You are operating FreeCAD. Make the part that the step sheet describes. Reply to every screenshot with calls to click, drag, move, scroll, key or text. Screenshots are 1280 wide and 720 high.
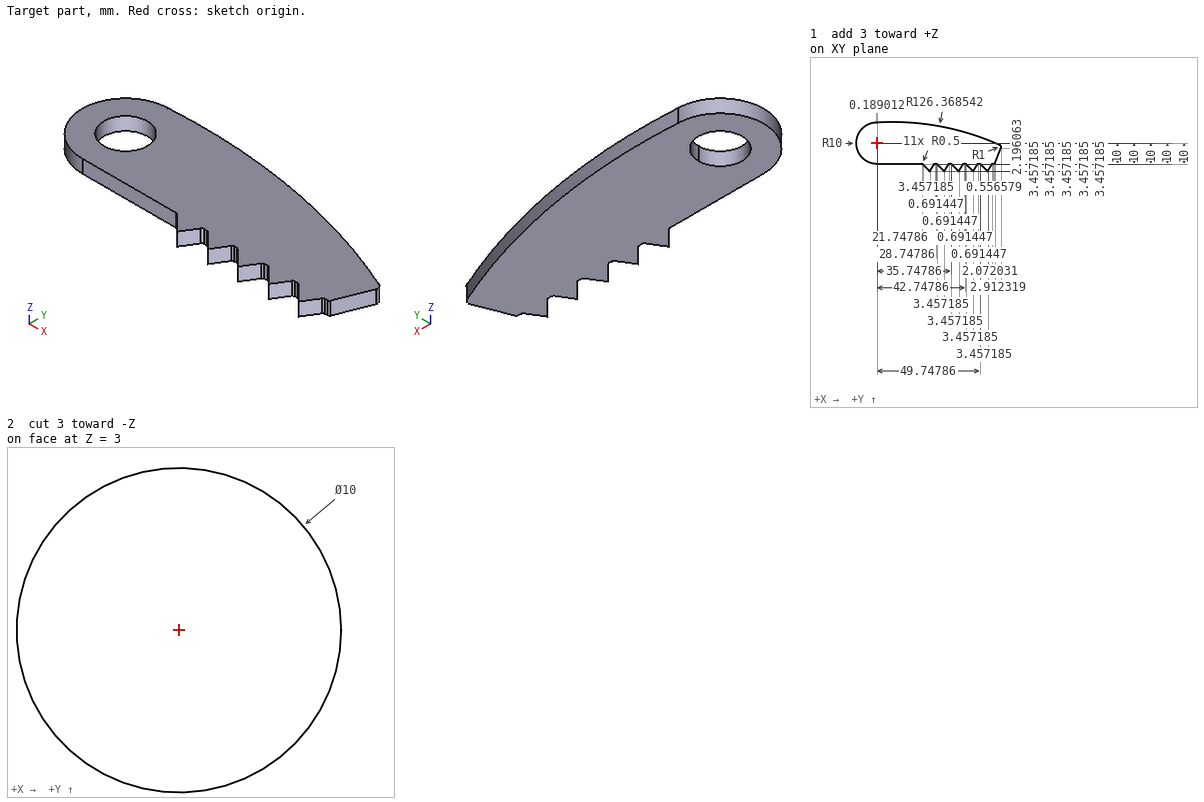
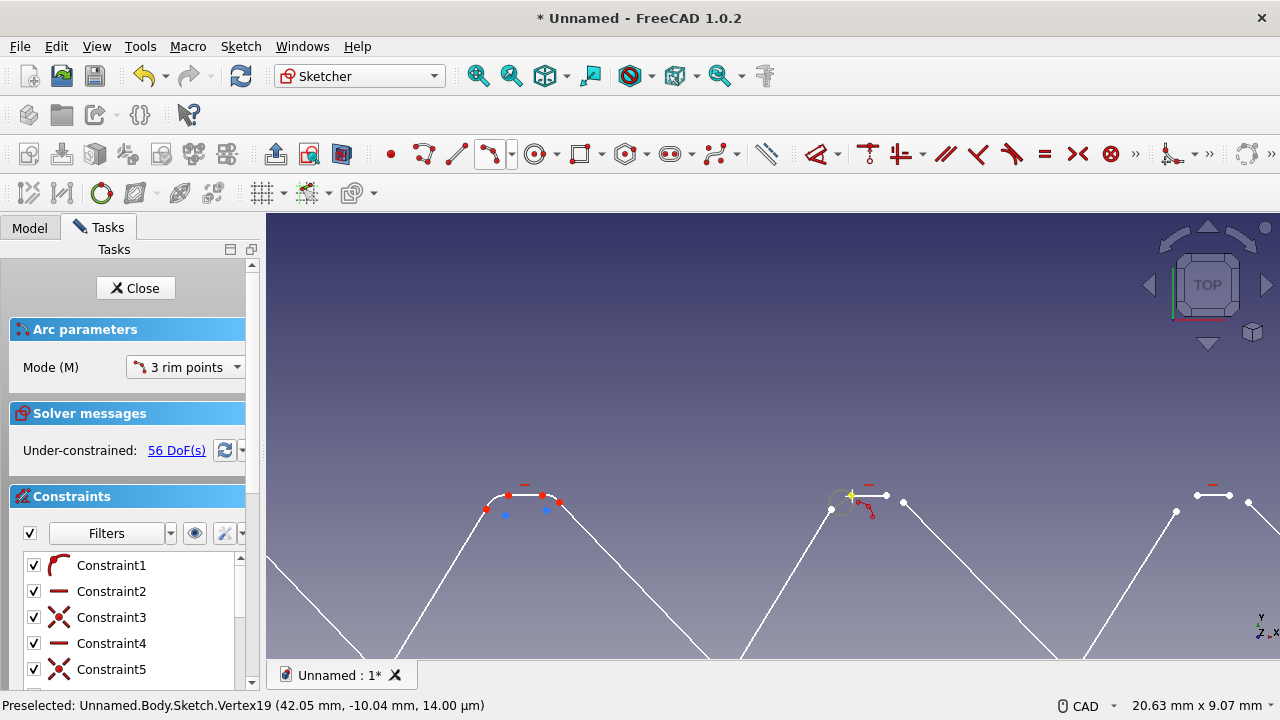
scroll(840, 497, up, 9)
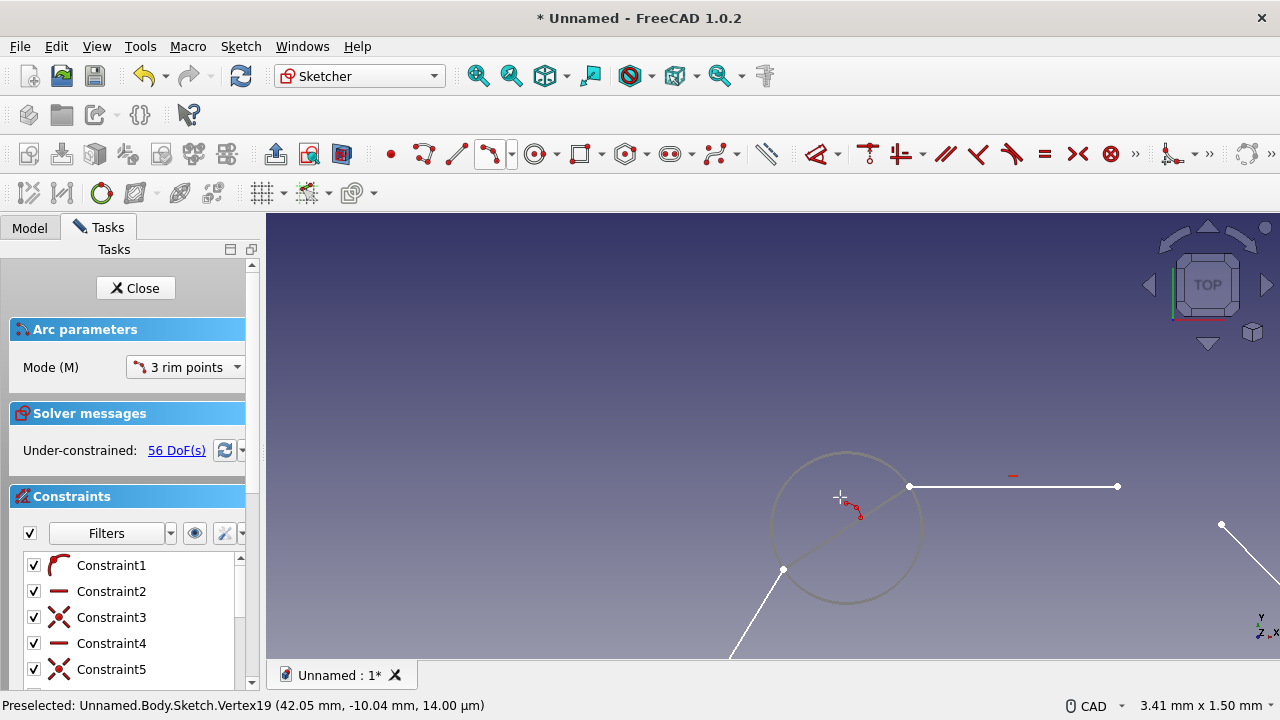
click(840, 495)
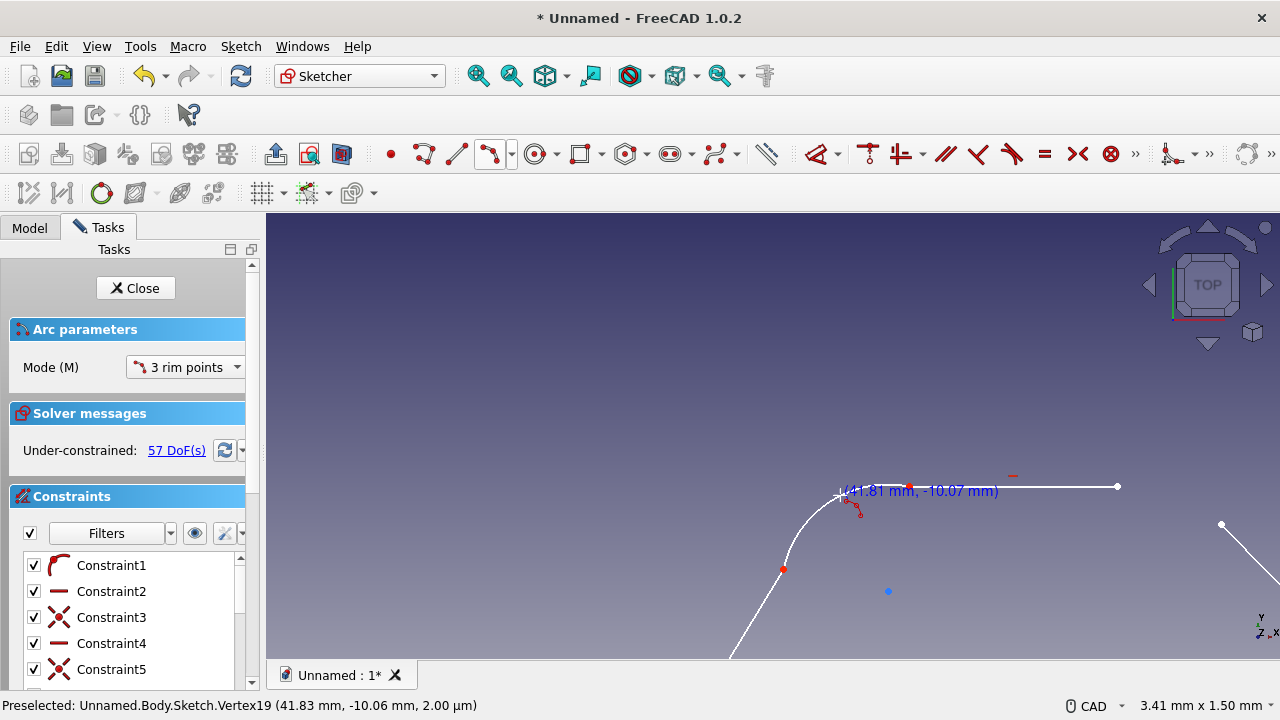
scroll(873, 519, down, 17)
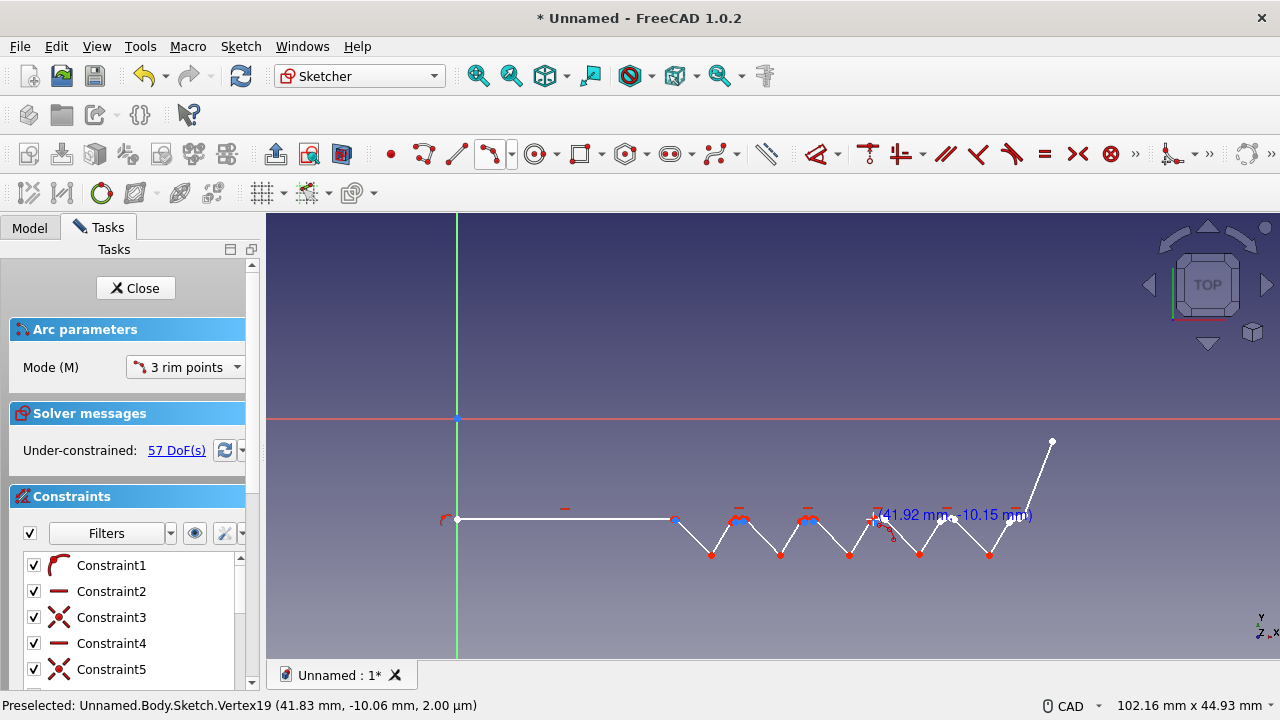
scroll(882, 518, up, 8)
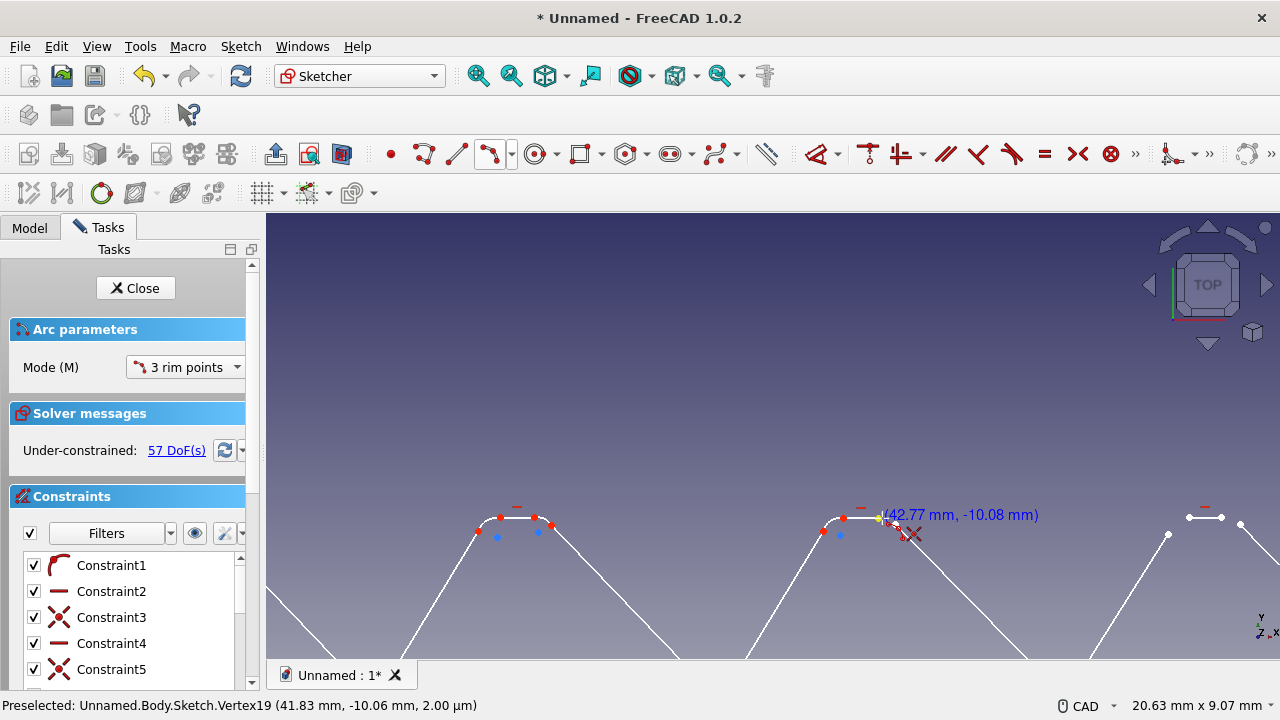
click(878, 518)
click(895, 524)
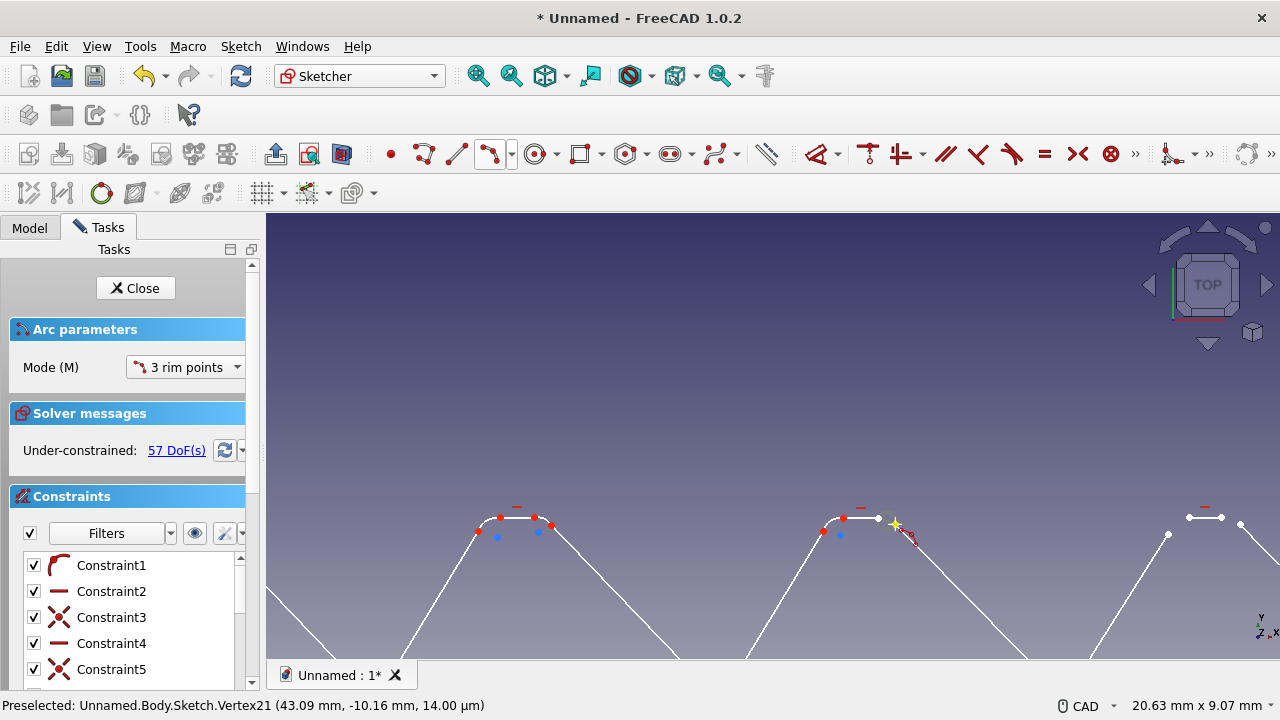
scroll(888, 518, up, 11)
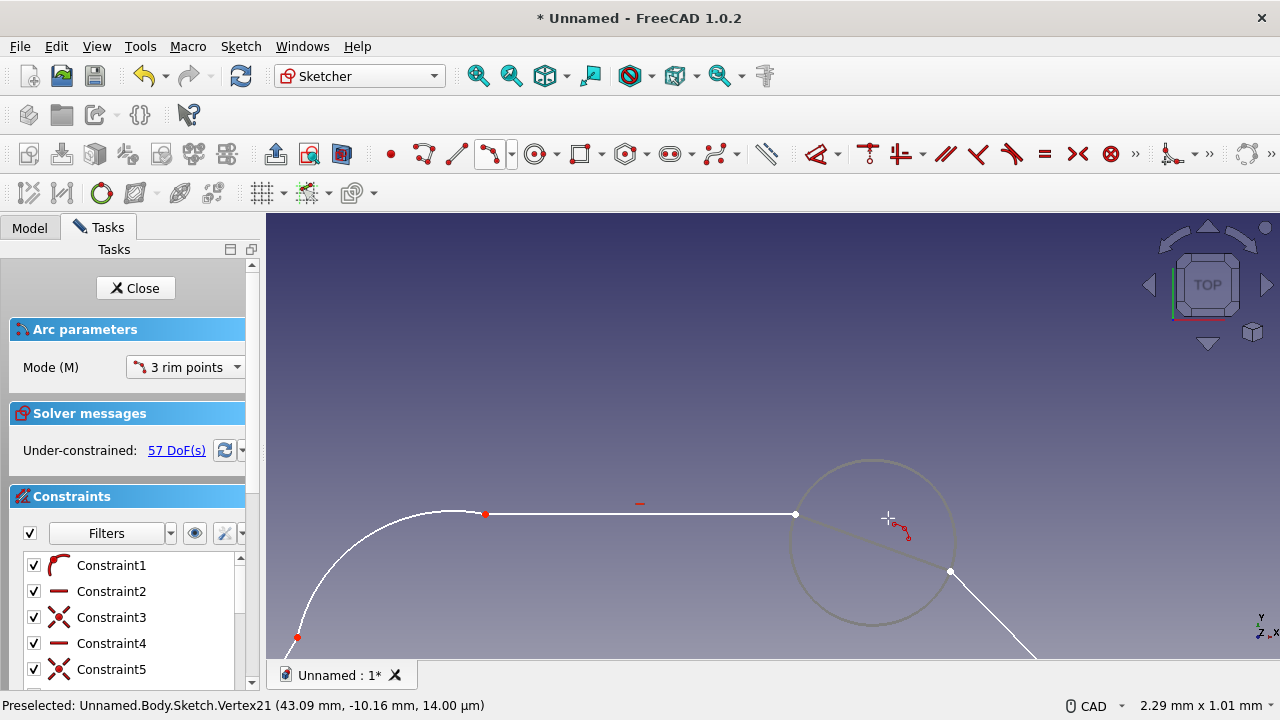
click(881, 516)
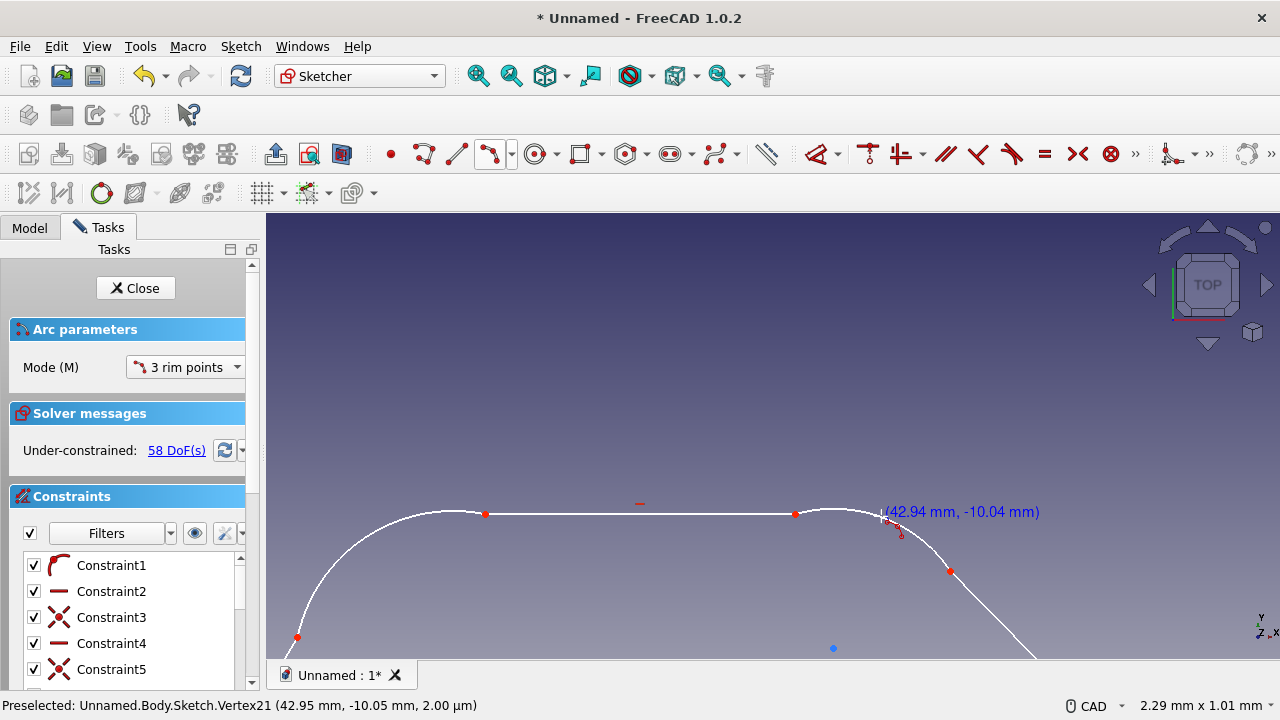
scroll(704, 436, down, 15)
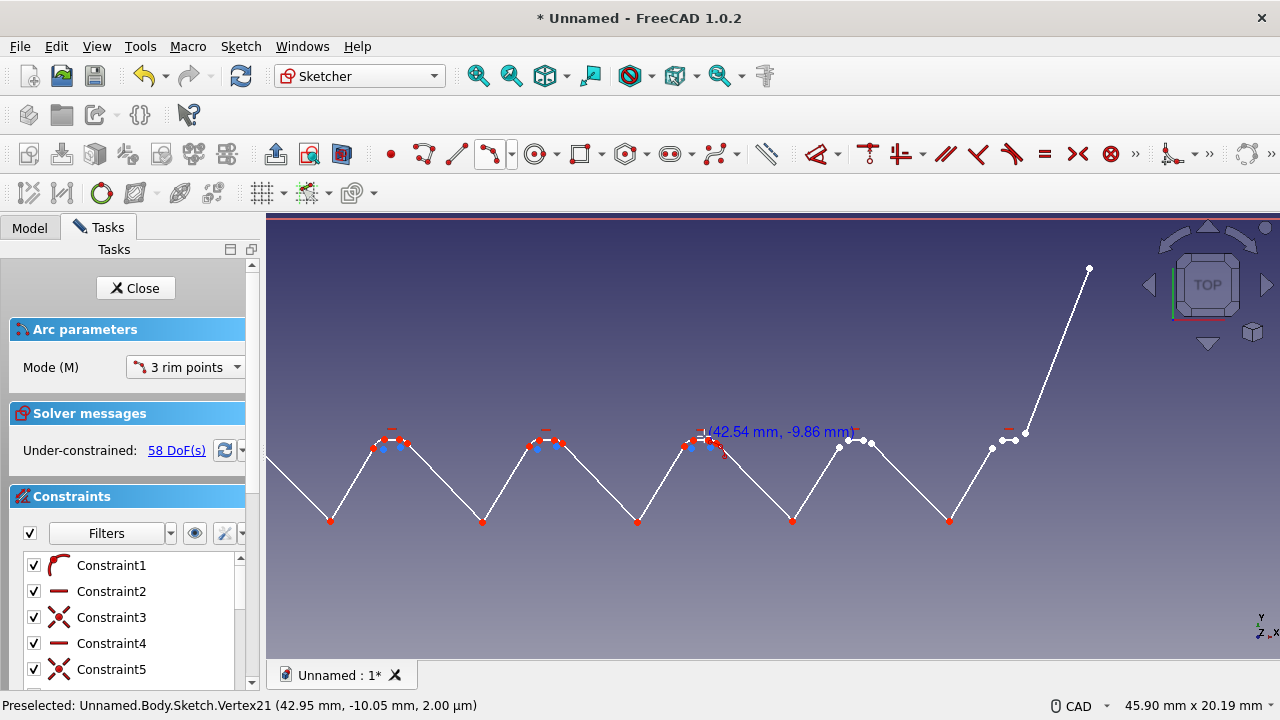
scroll(930, 539, down, 5)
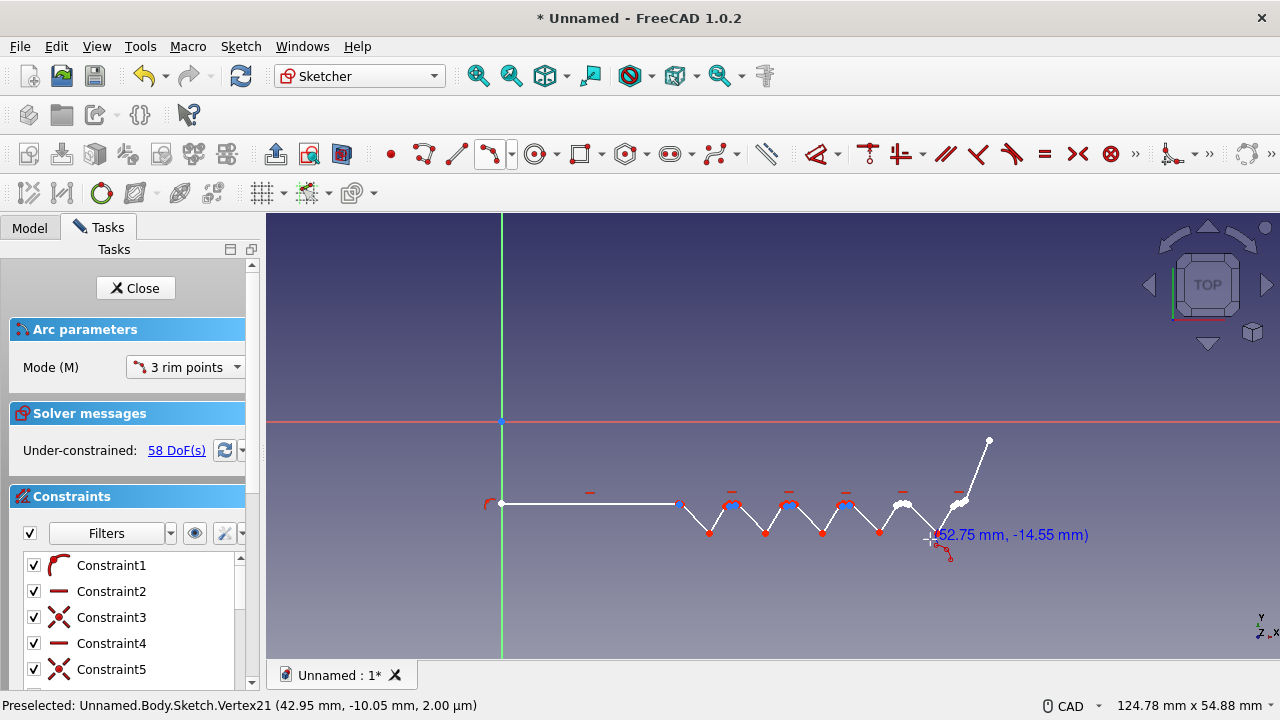
scroll(897, 505, up, 7)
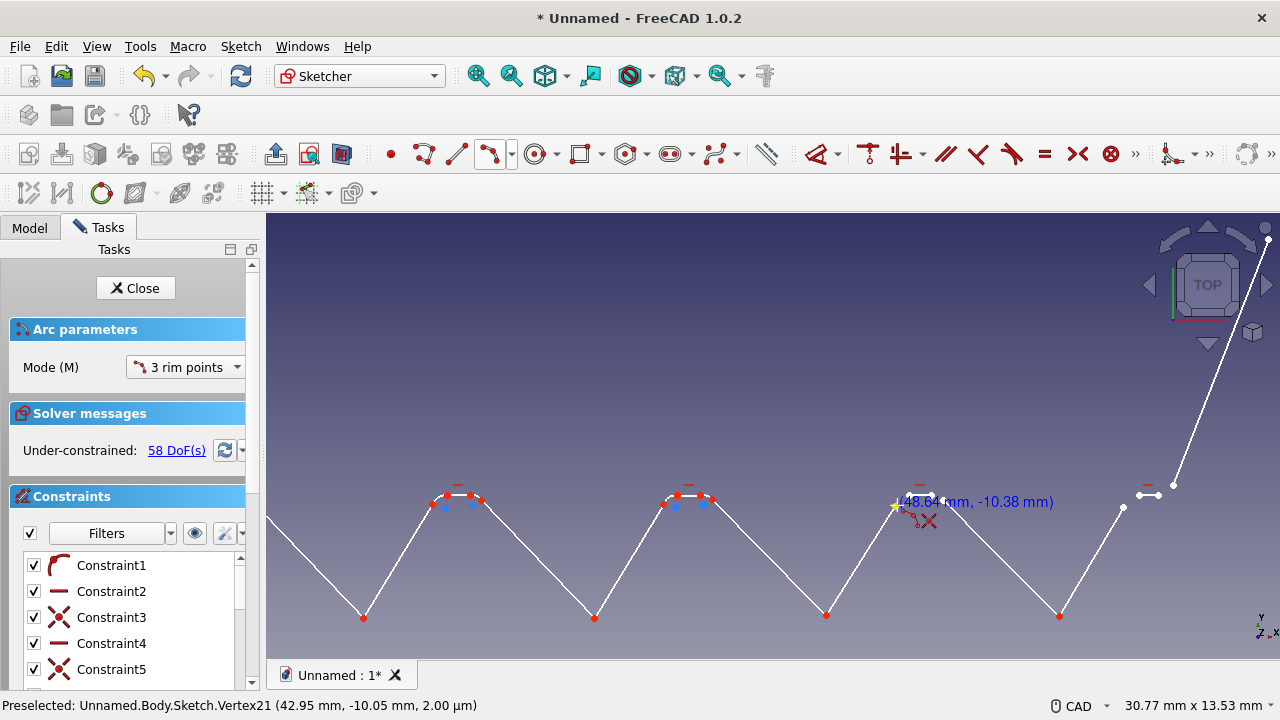
click(895, 506)